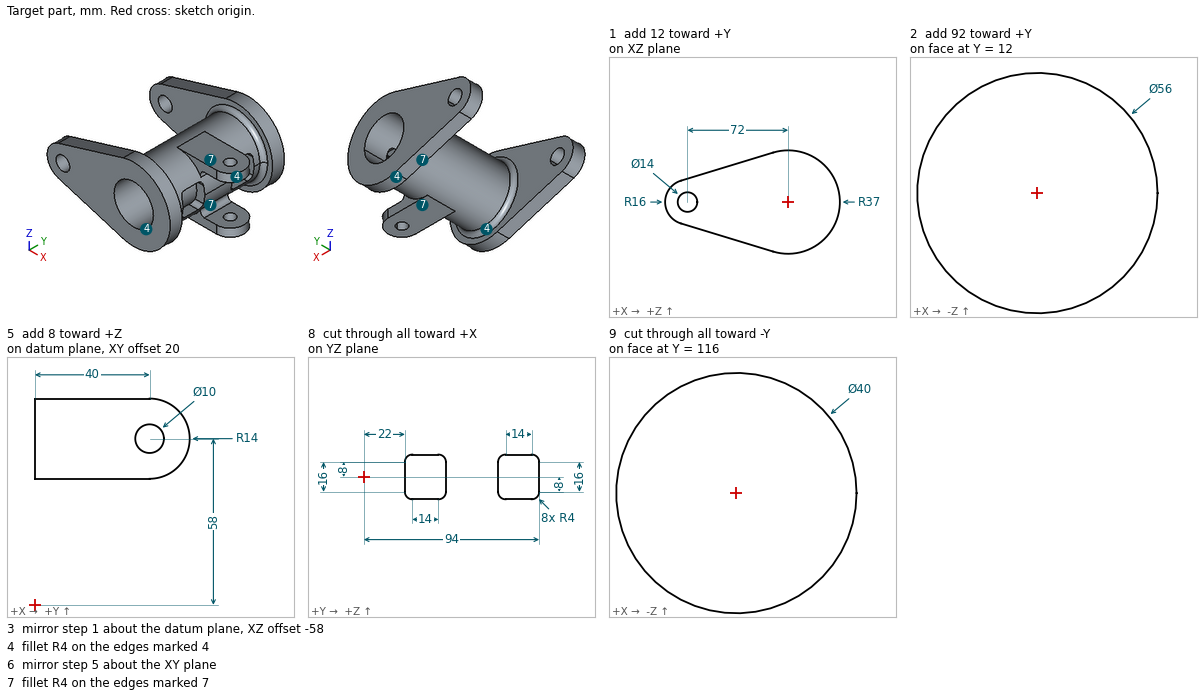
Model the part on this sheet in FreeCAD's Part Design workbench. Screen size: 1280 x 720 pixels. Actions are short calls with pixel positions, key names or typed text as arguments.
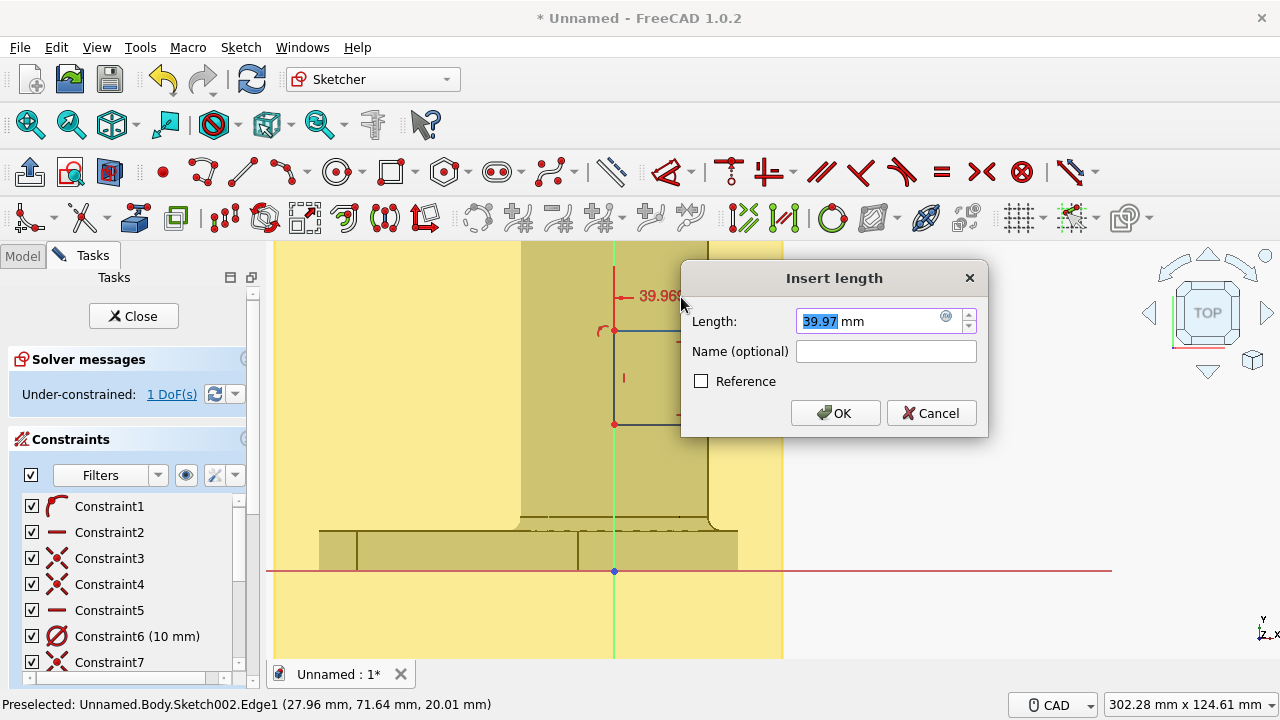
text(40)
key(Return)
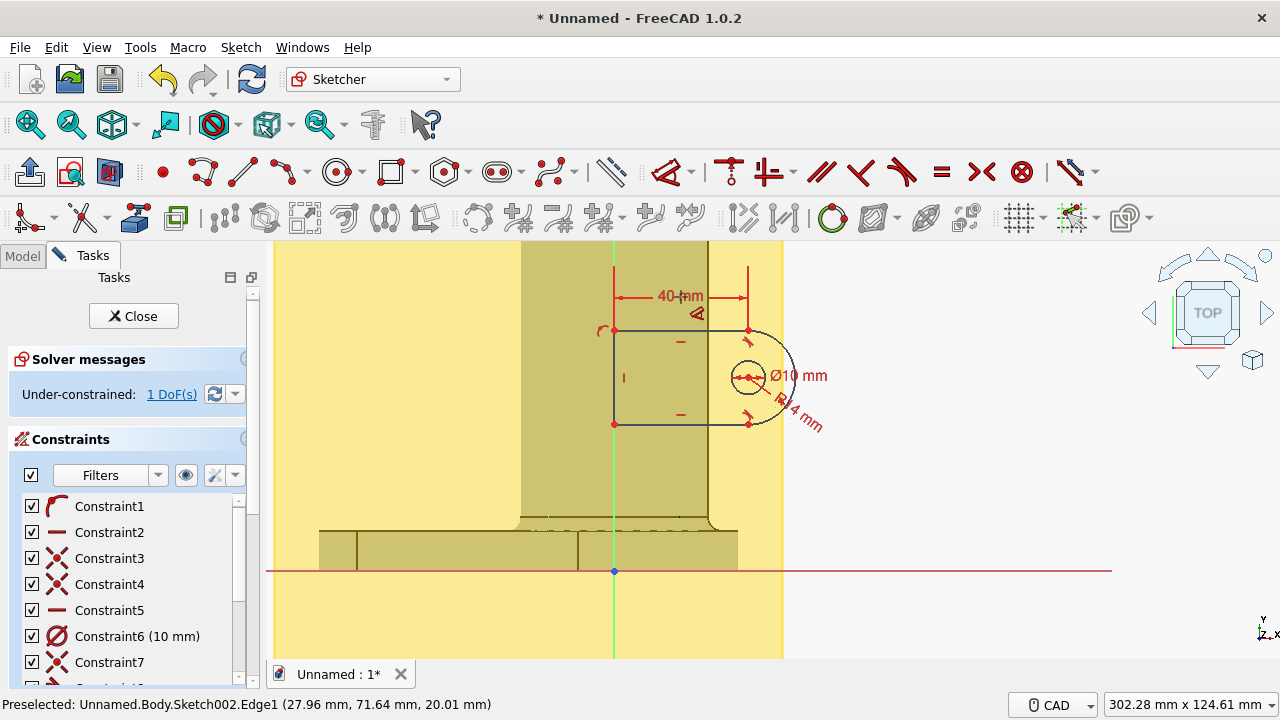
click(748, 378)
click(580, 474)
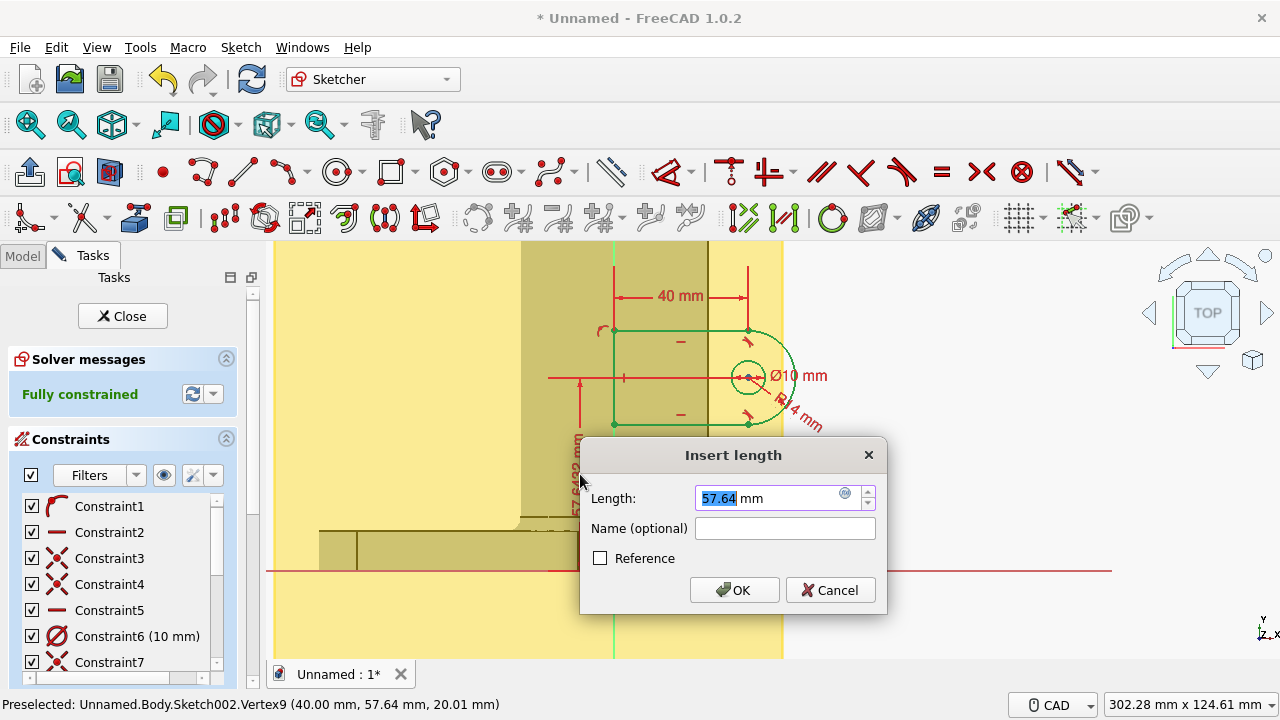
text(58)
key(Return)
key(Escape)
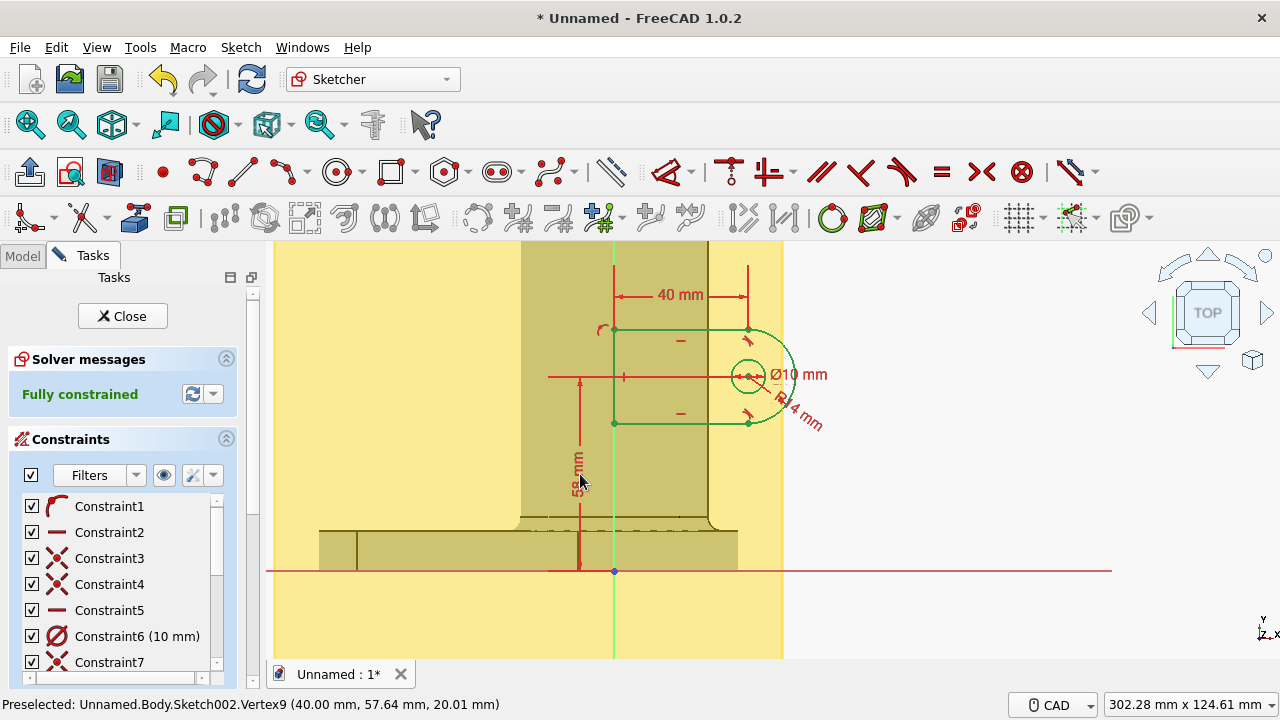
click(123, 316)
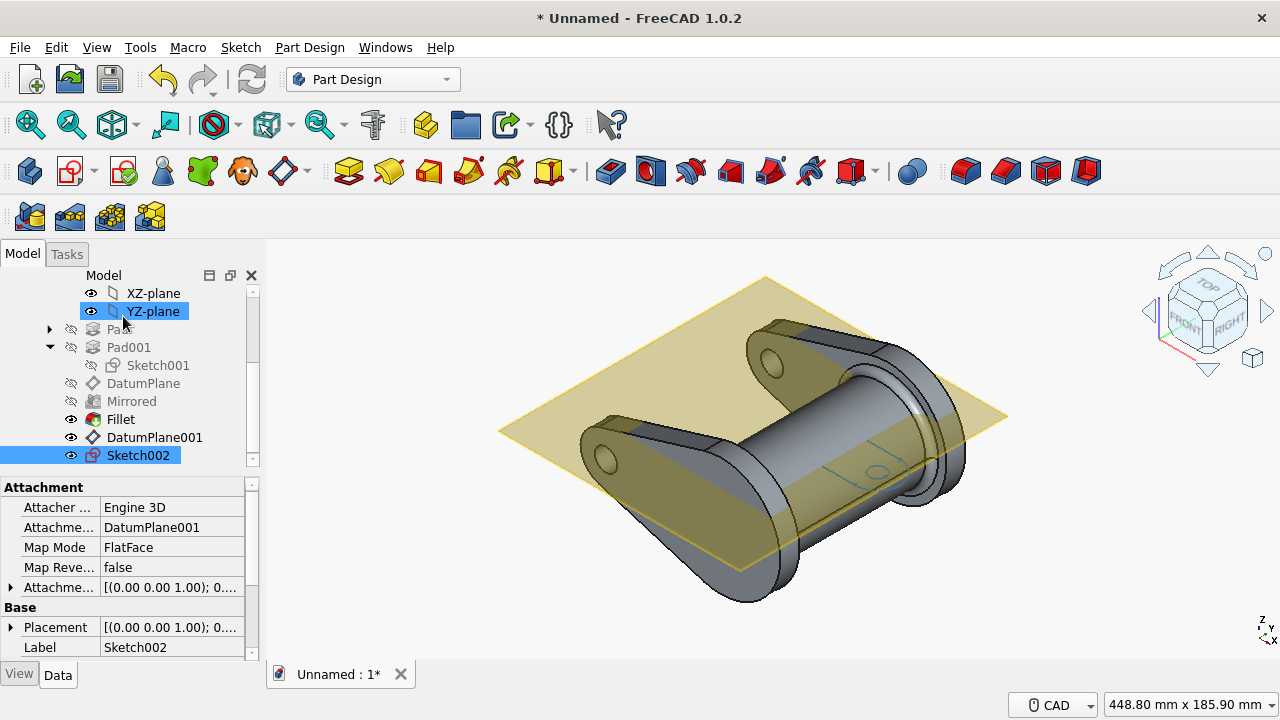
click(350, 172)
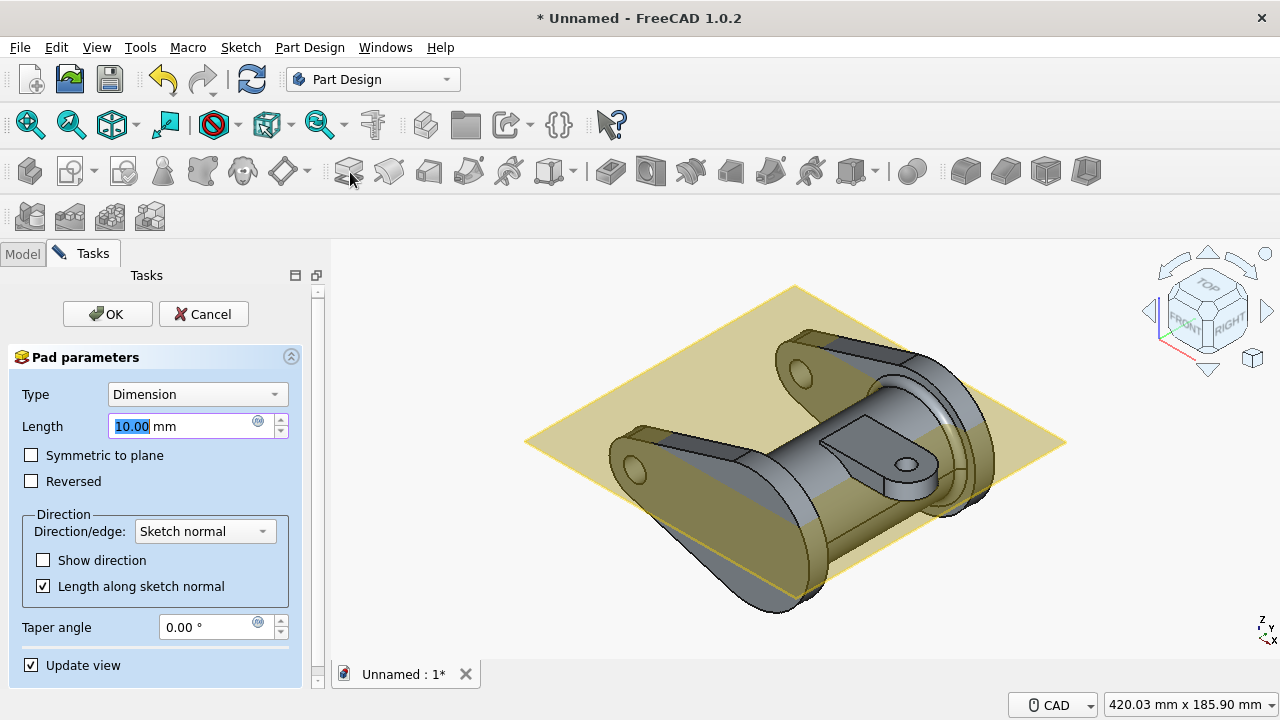
text(8)
key(Tab)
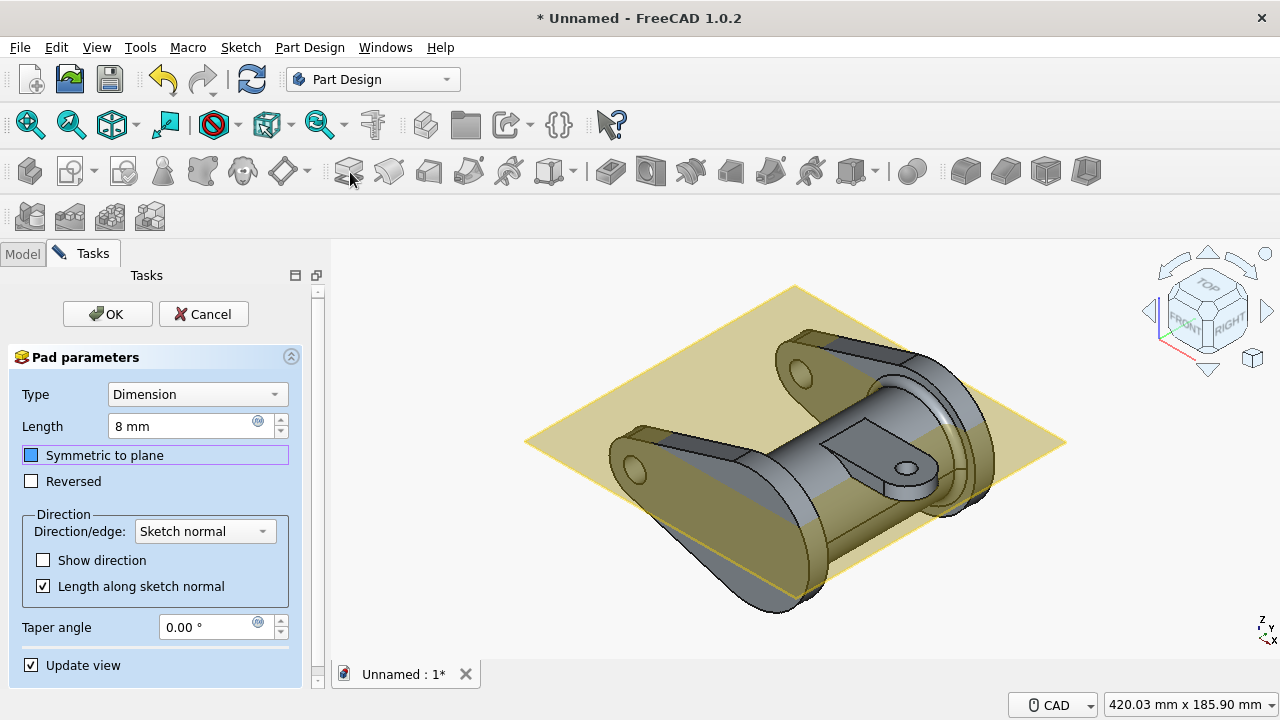
click(108, 314)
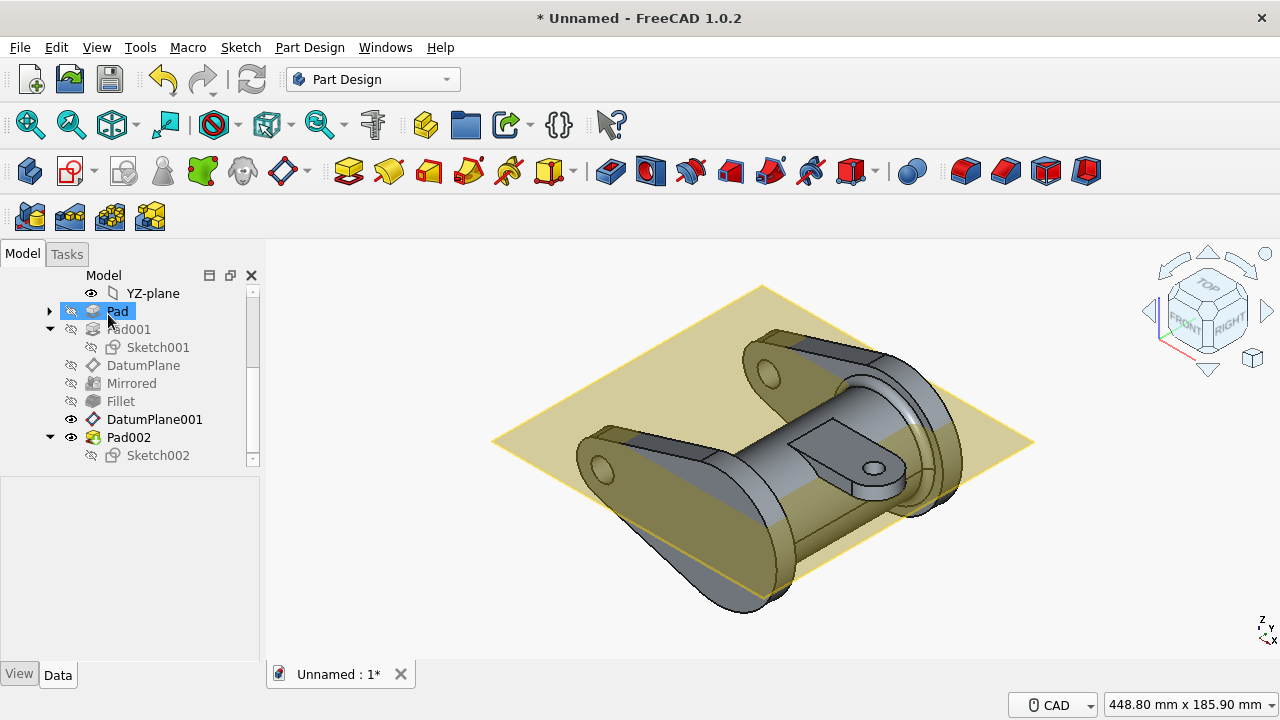
click(116, 419)
key(space)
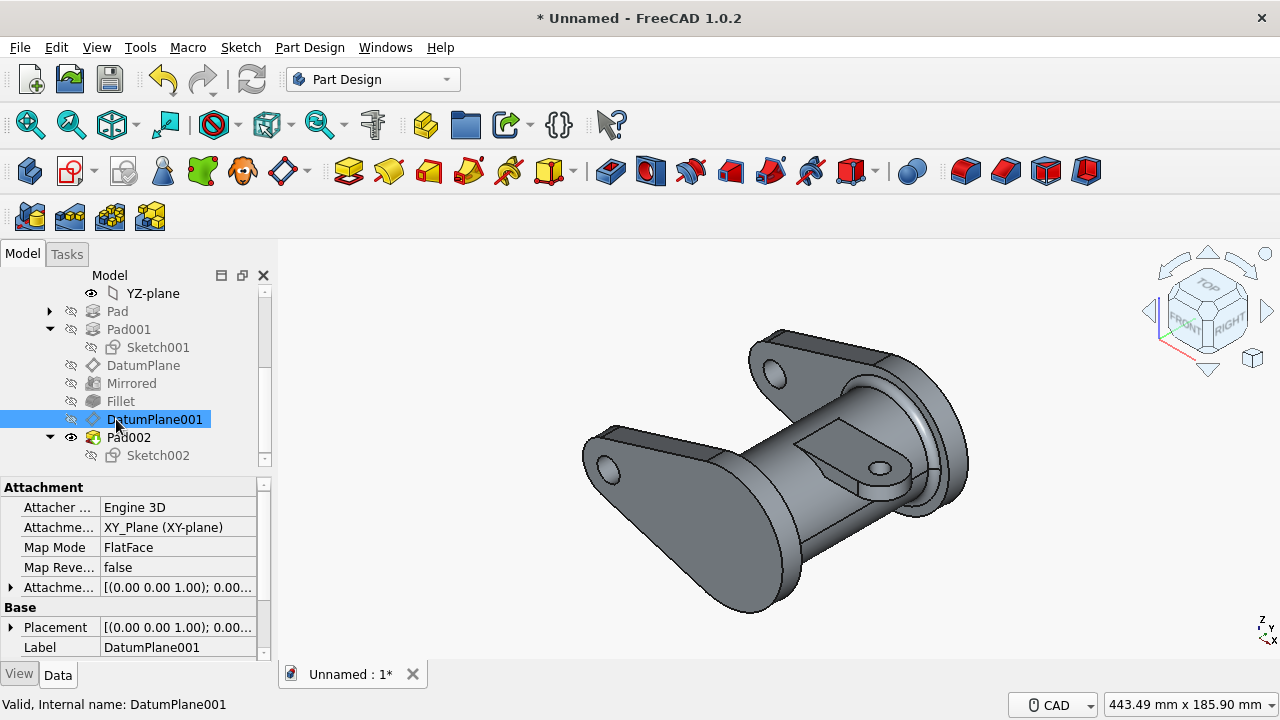
click(116, 437)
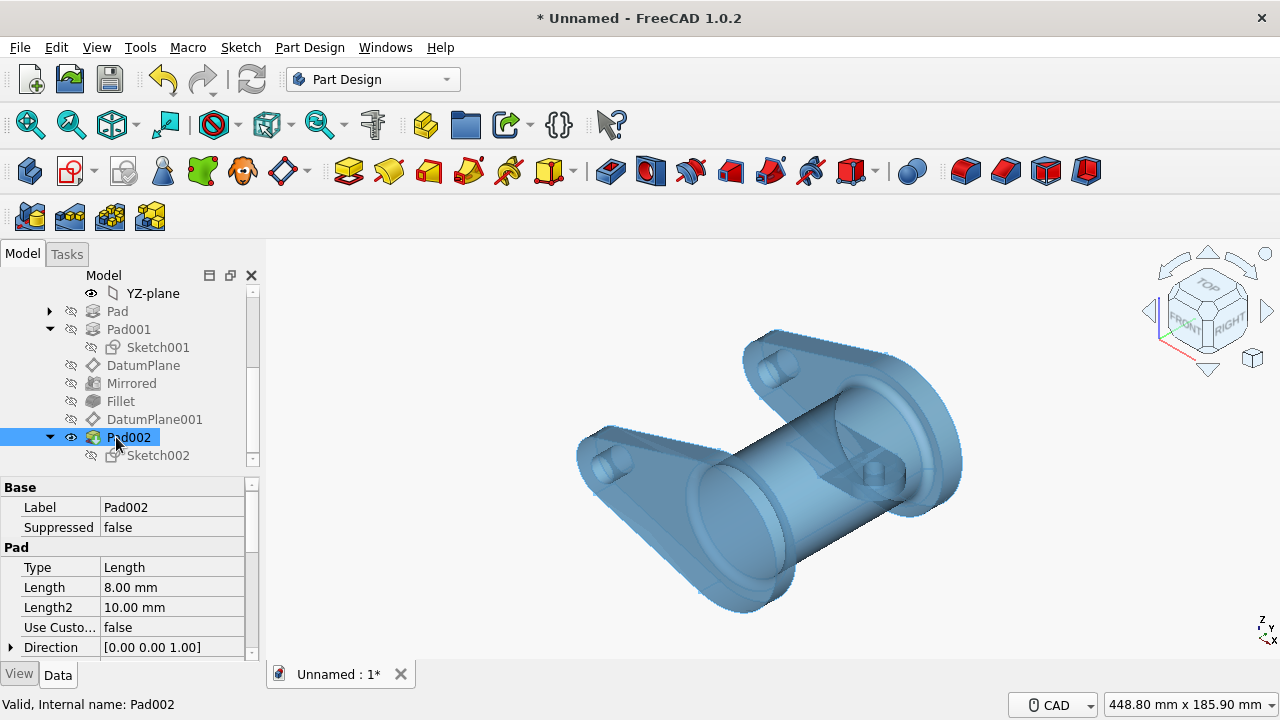
click(30, 216)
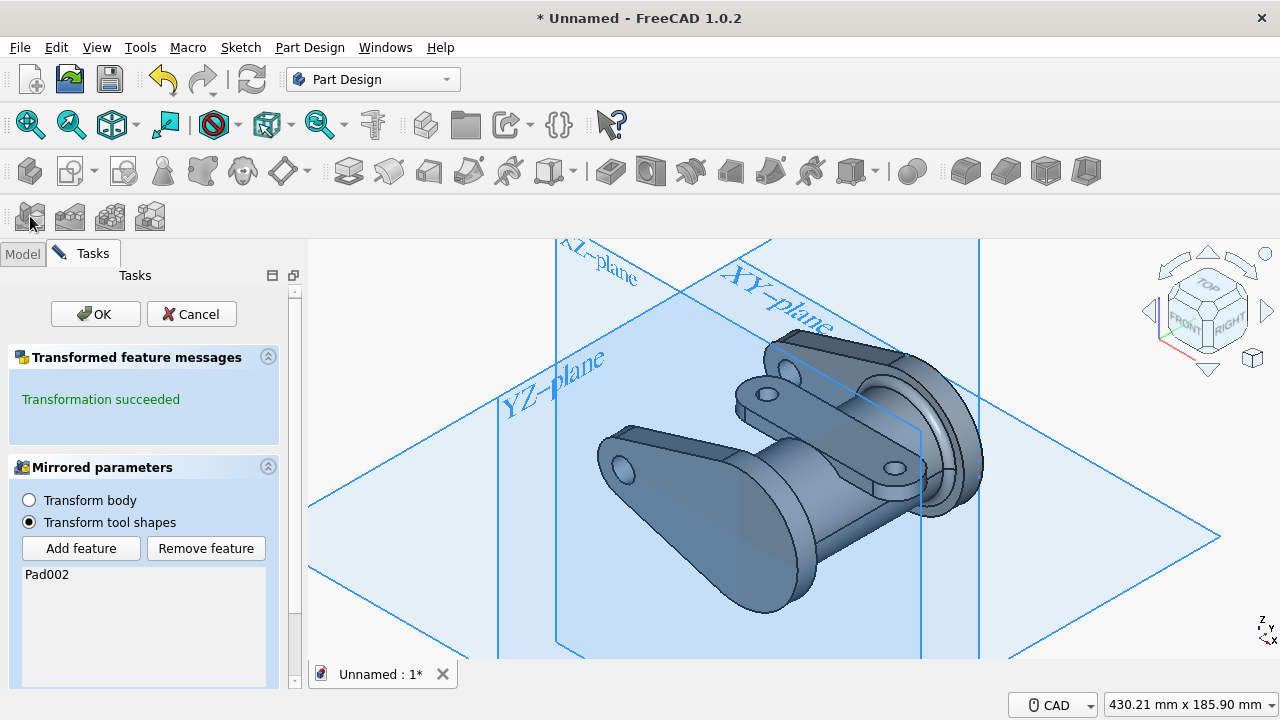
scroll(295, 486, down, 2)